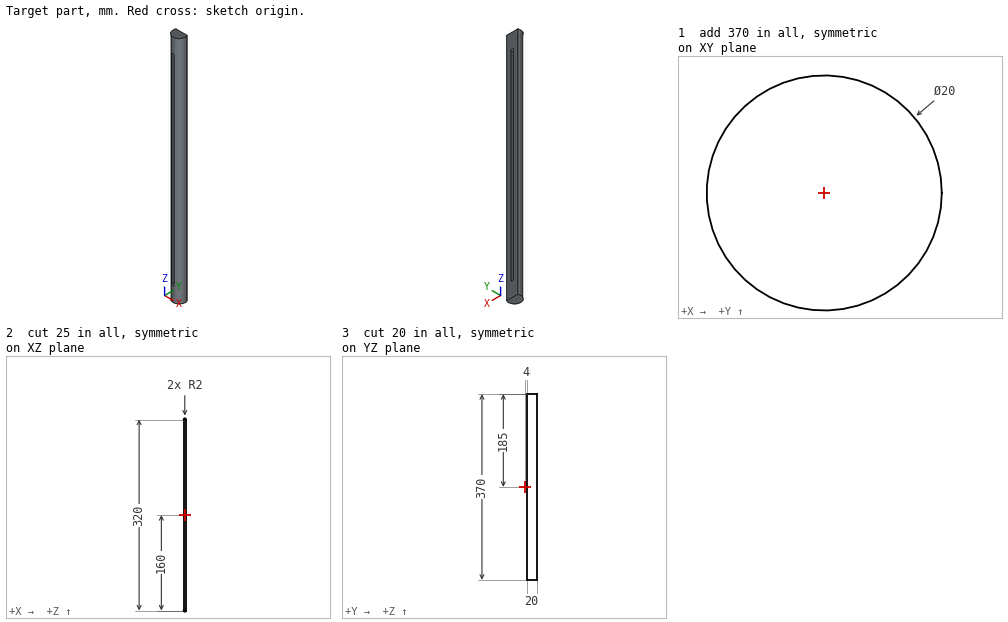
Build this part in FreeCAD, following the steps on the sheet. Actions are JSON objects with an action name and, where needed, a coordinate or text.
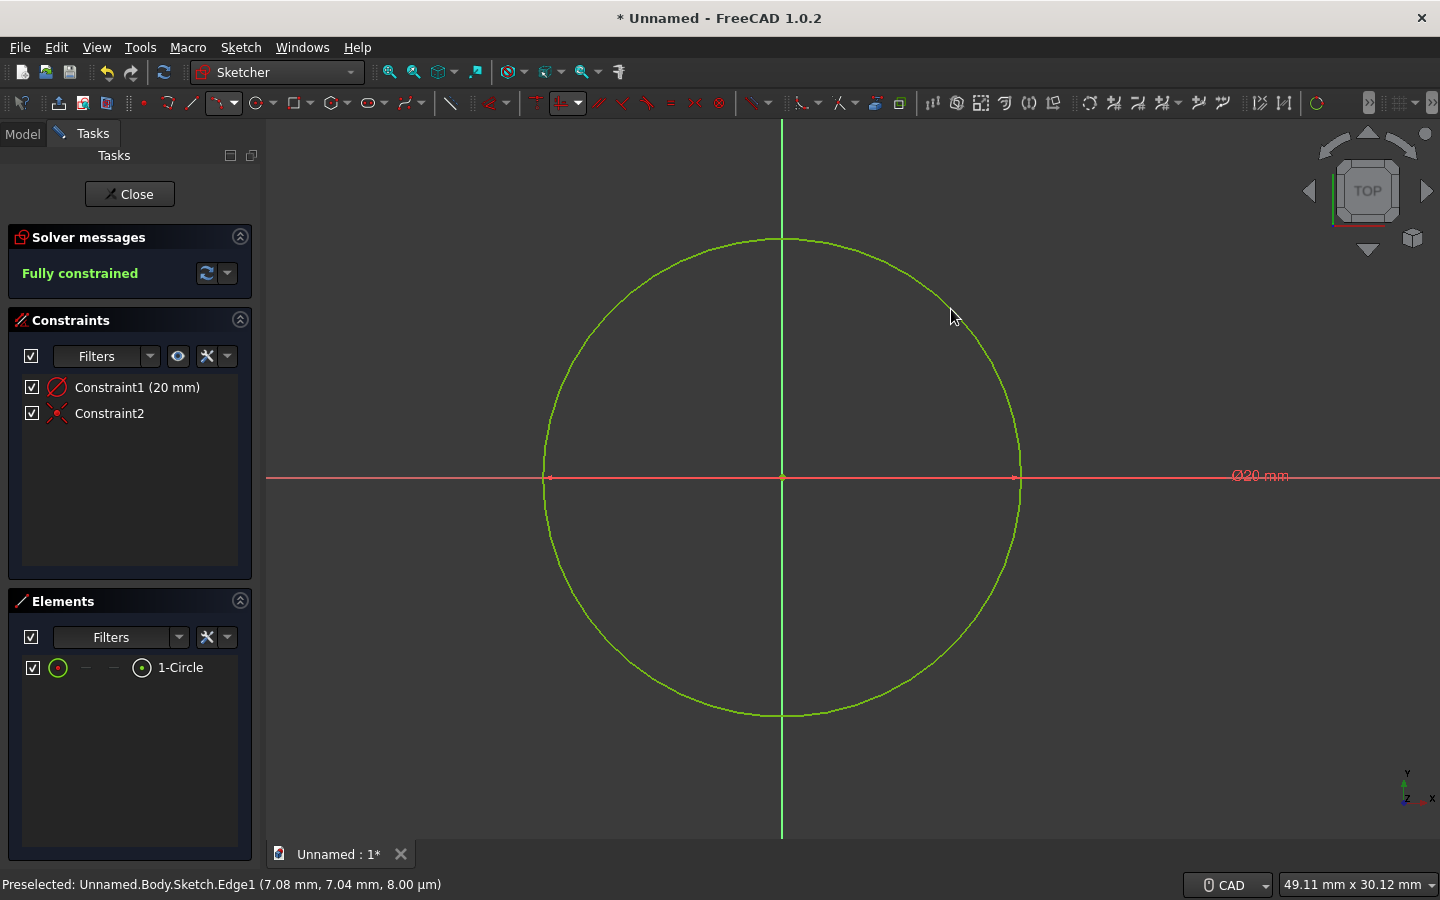
{"action": "left_click", "coordinate": [130, 194]}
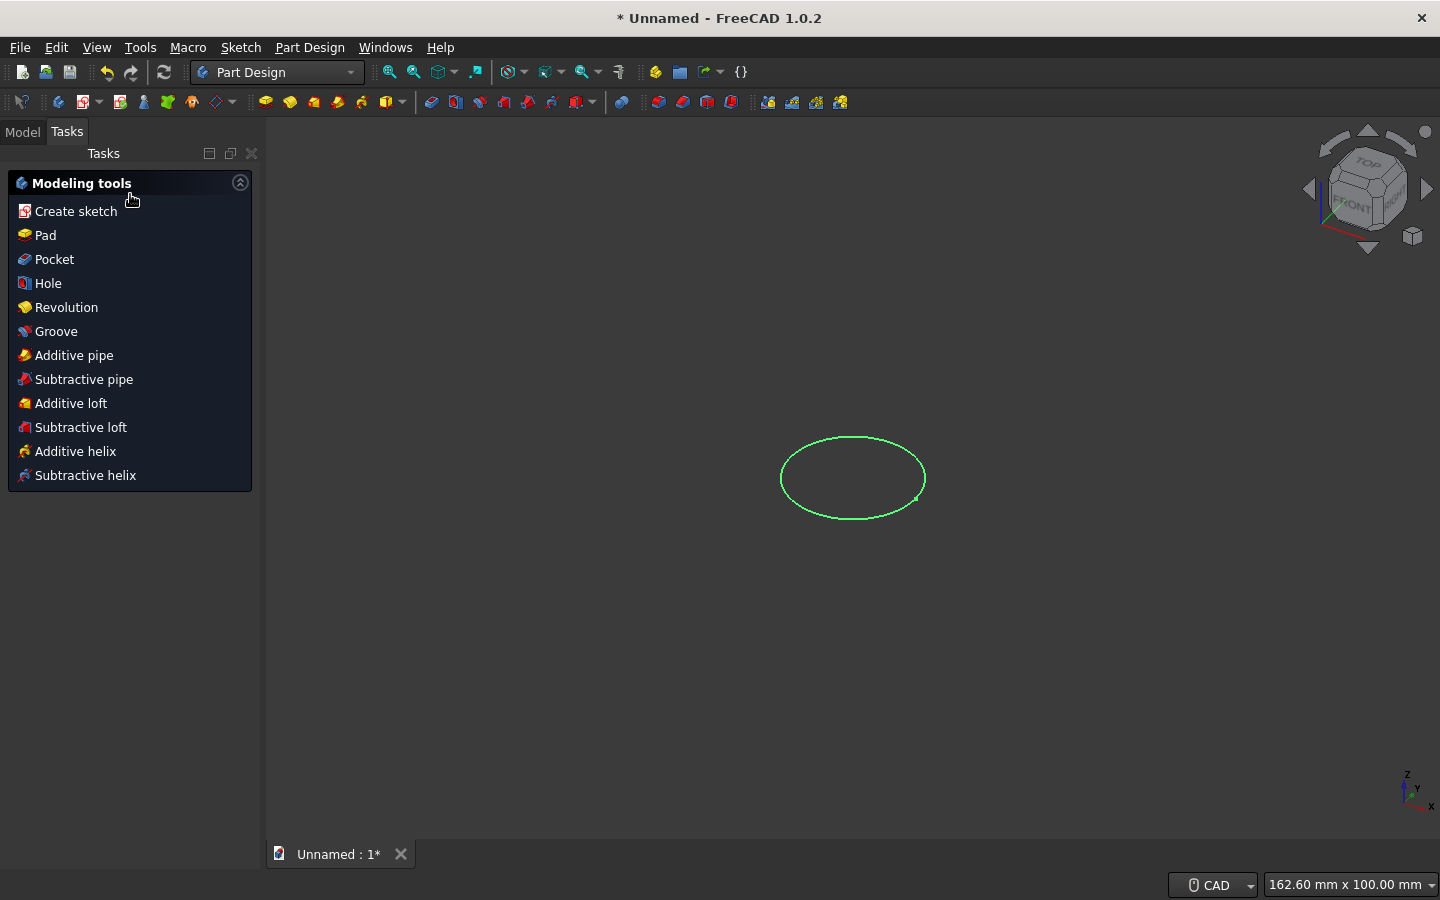
{"action": "left_click", "coordinate": [266, 102]}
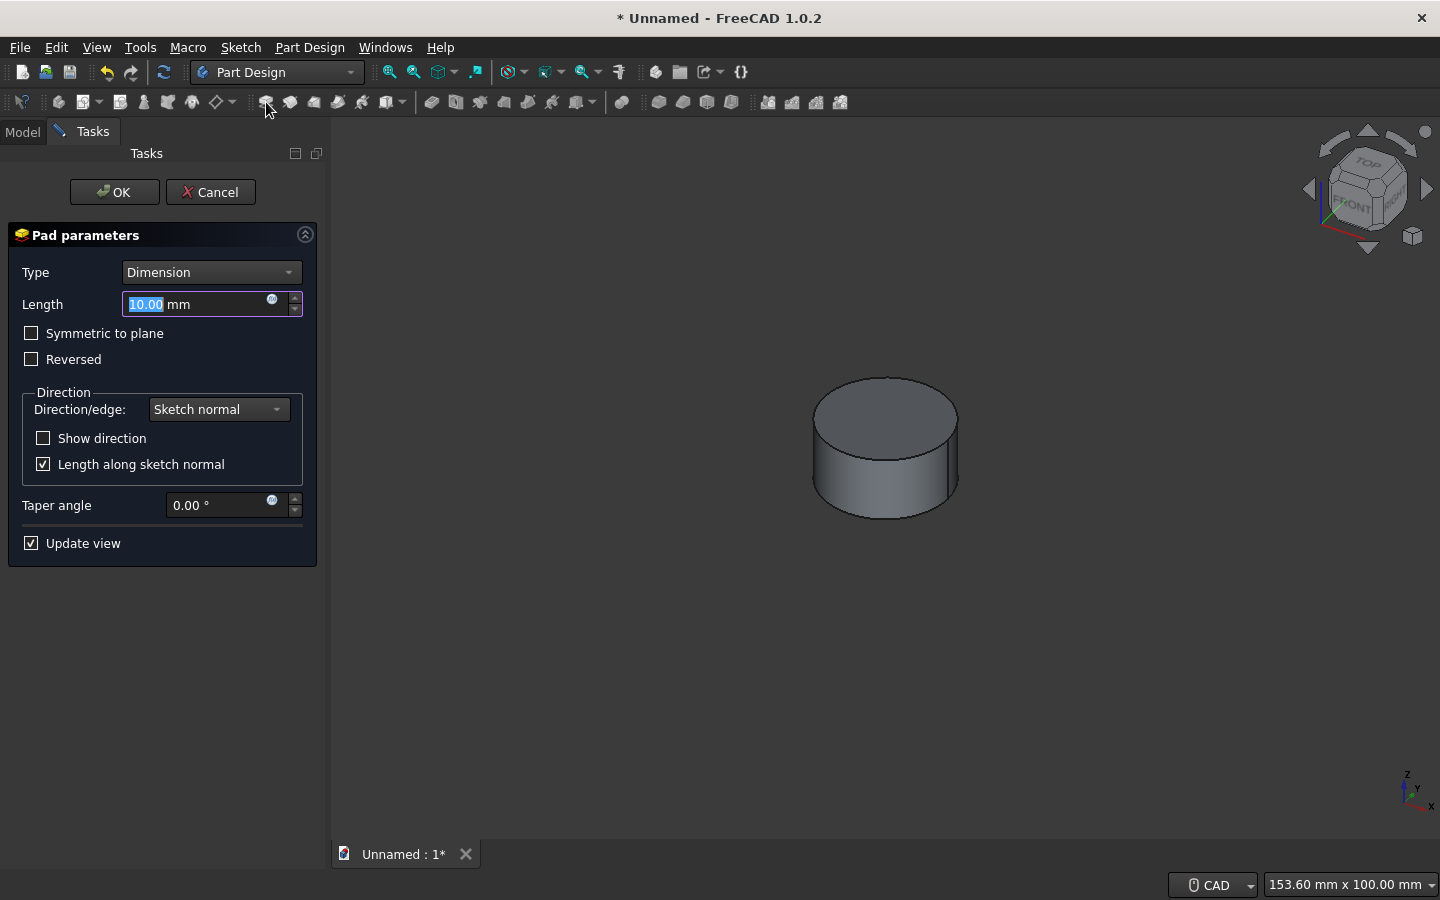
{"action": "type", "text": "370"}
{"action": "key", "text": "Tab"}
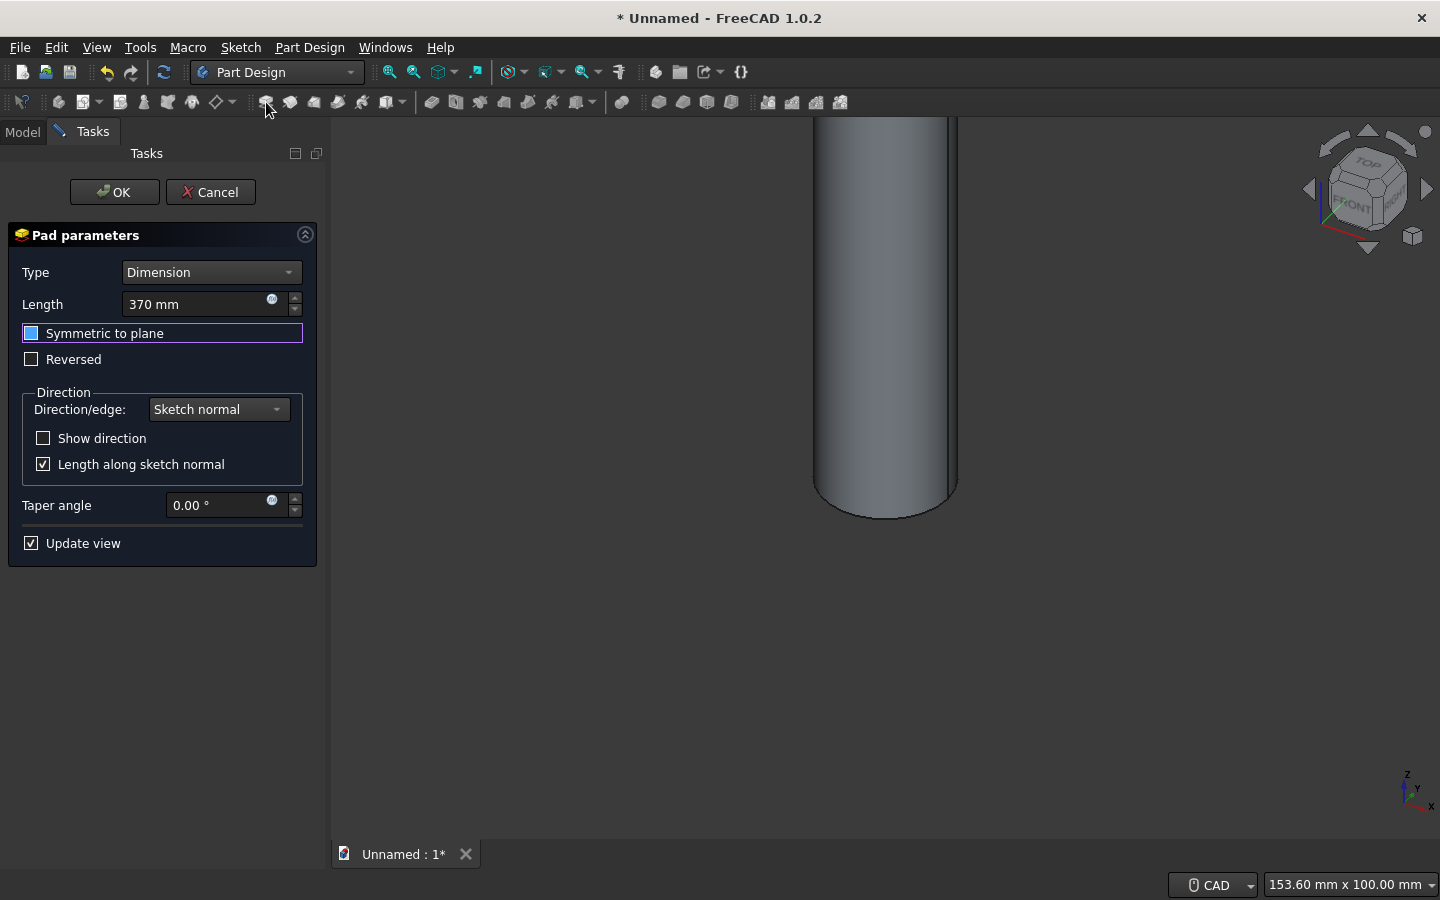
{"action": "left_click", "coordinate": [30, 333]}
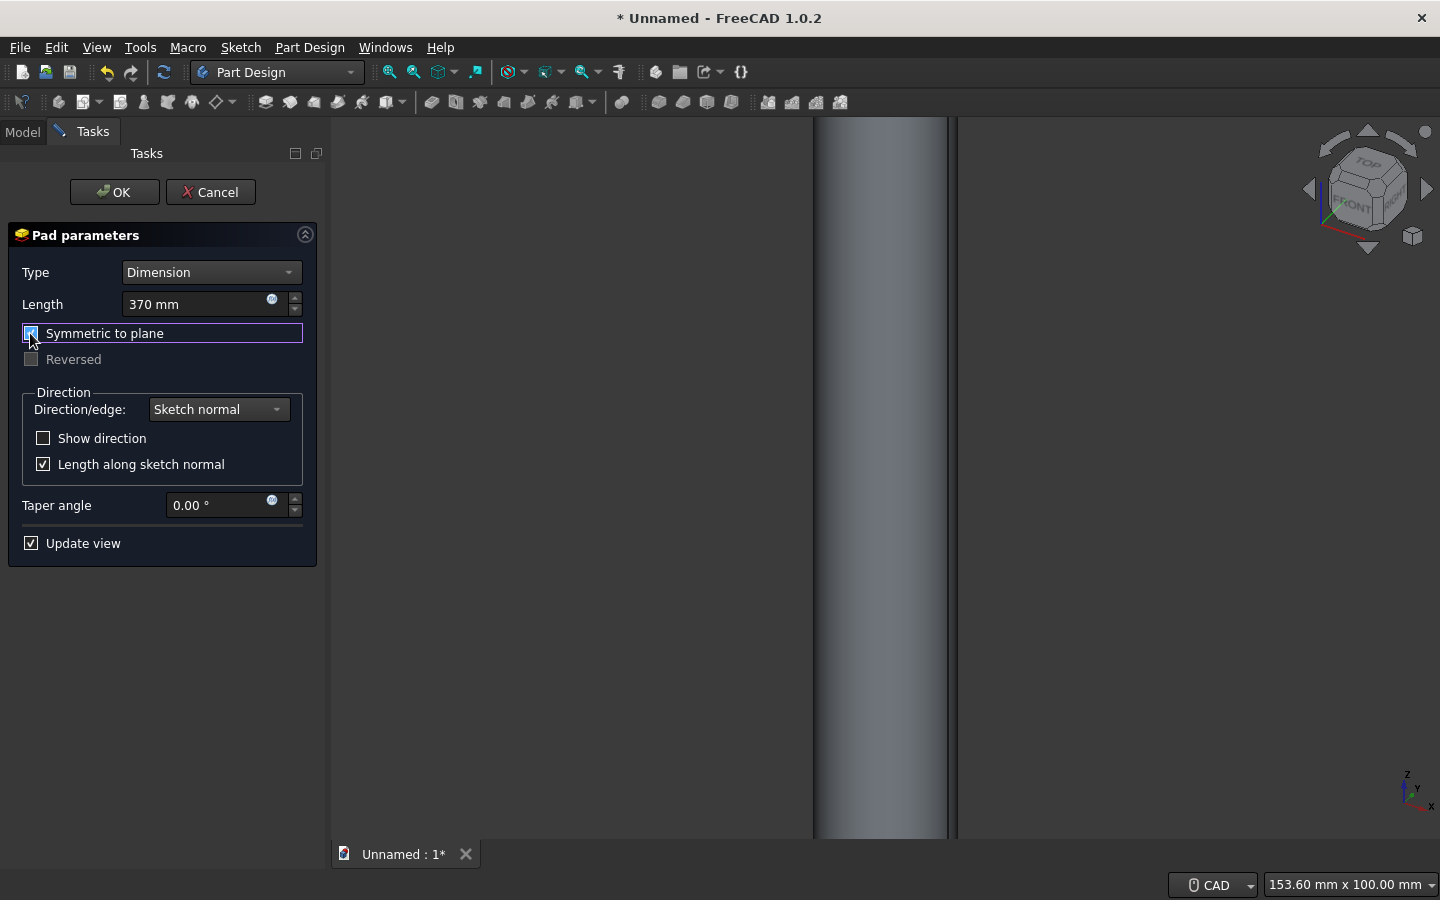
{"action": "left_click", "coordinate": [115, 192]}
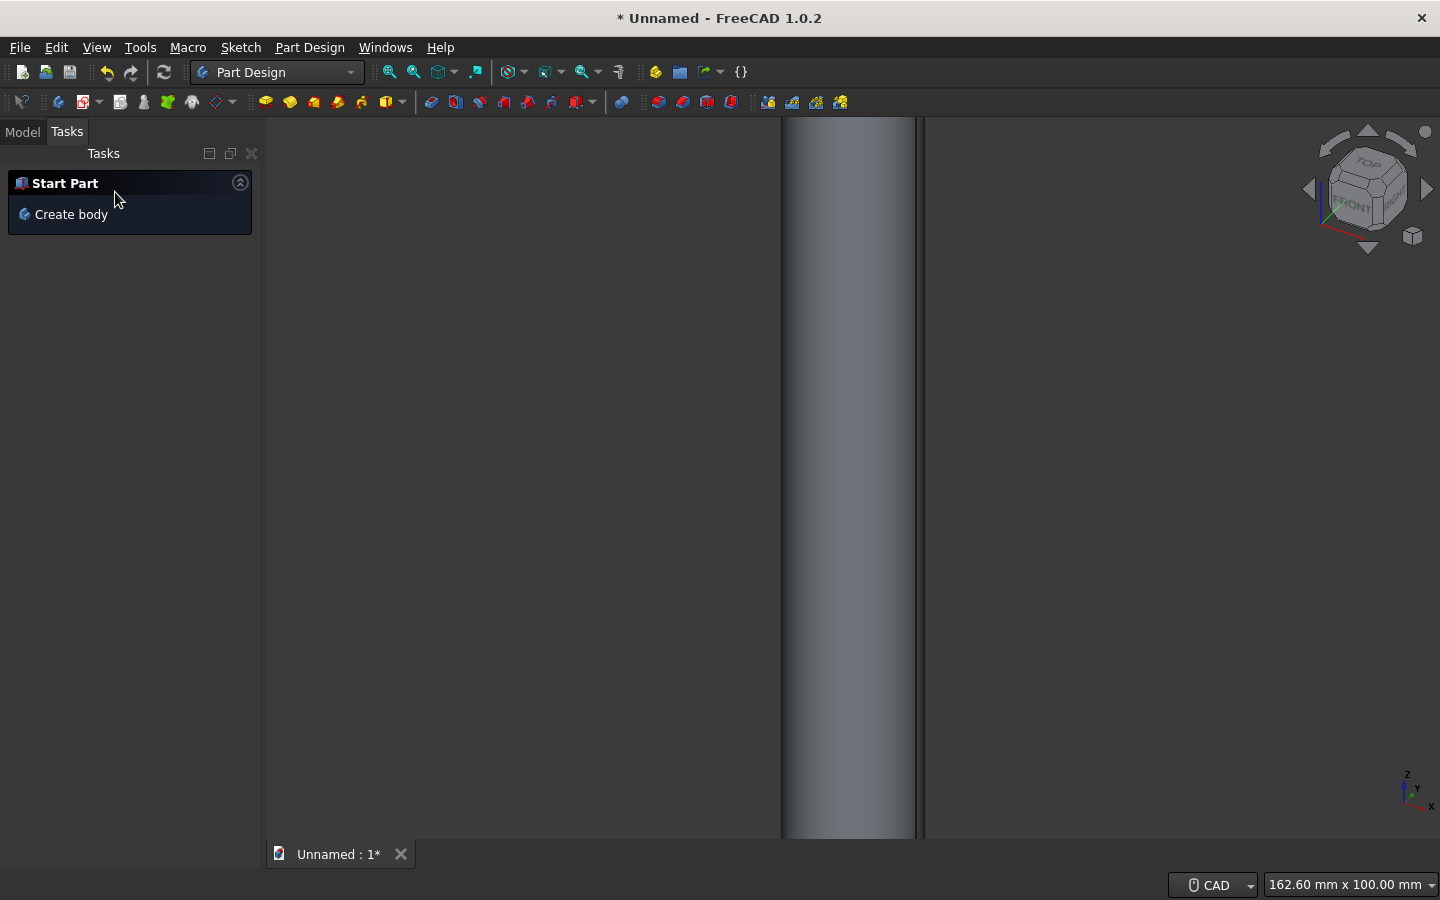
{"action": "left_click", "coordinate": [390, 72]}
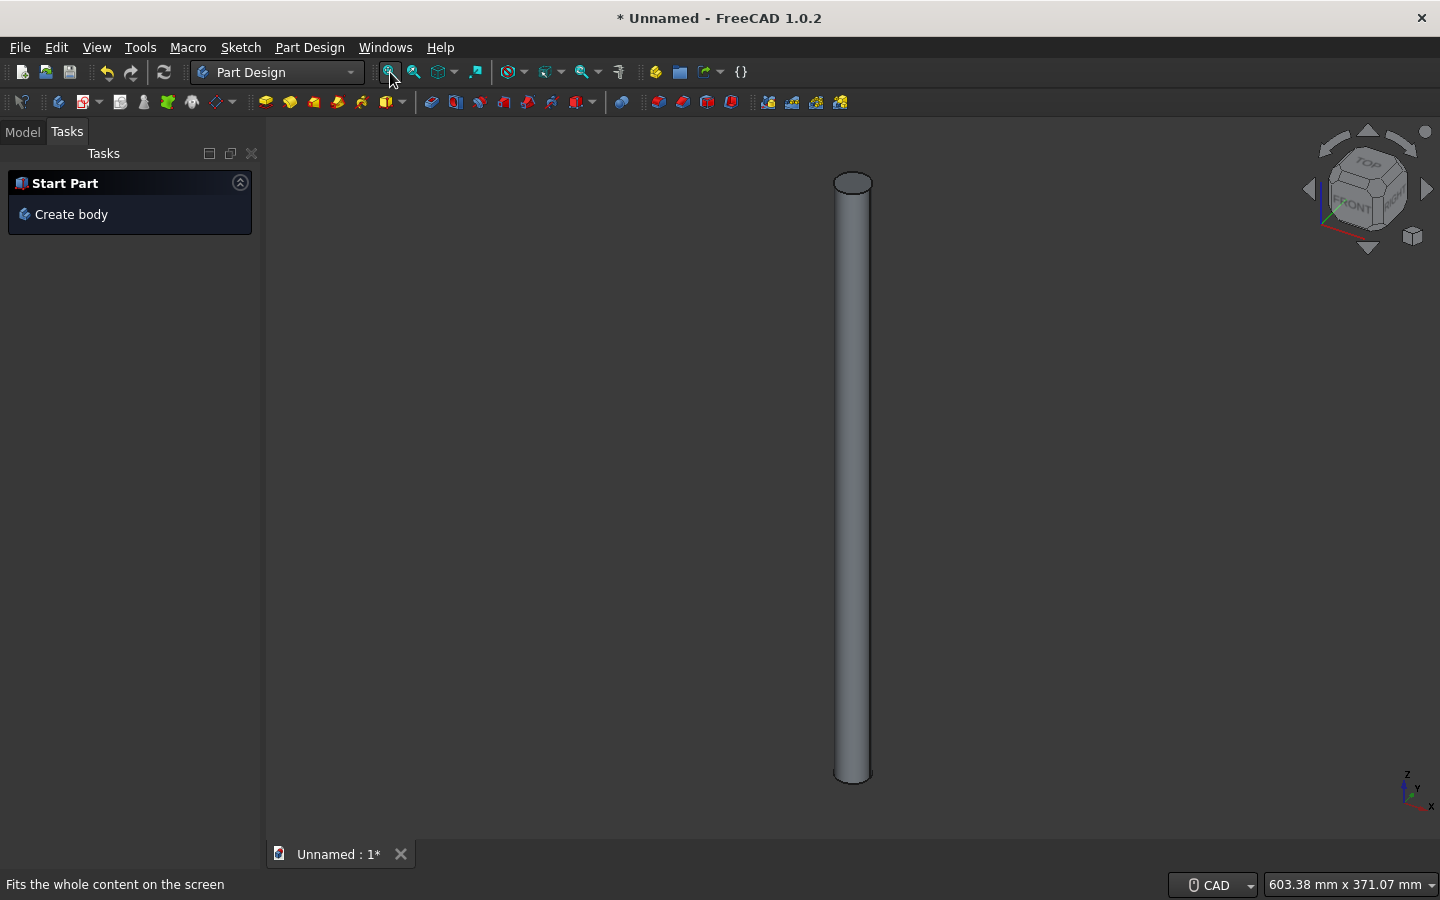
{"action": "left_click", "coordinate": [84, 102]}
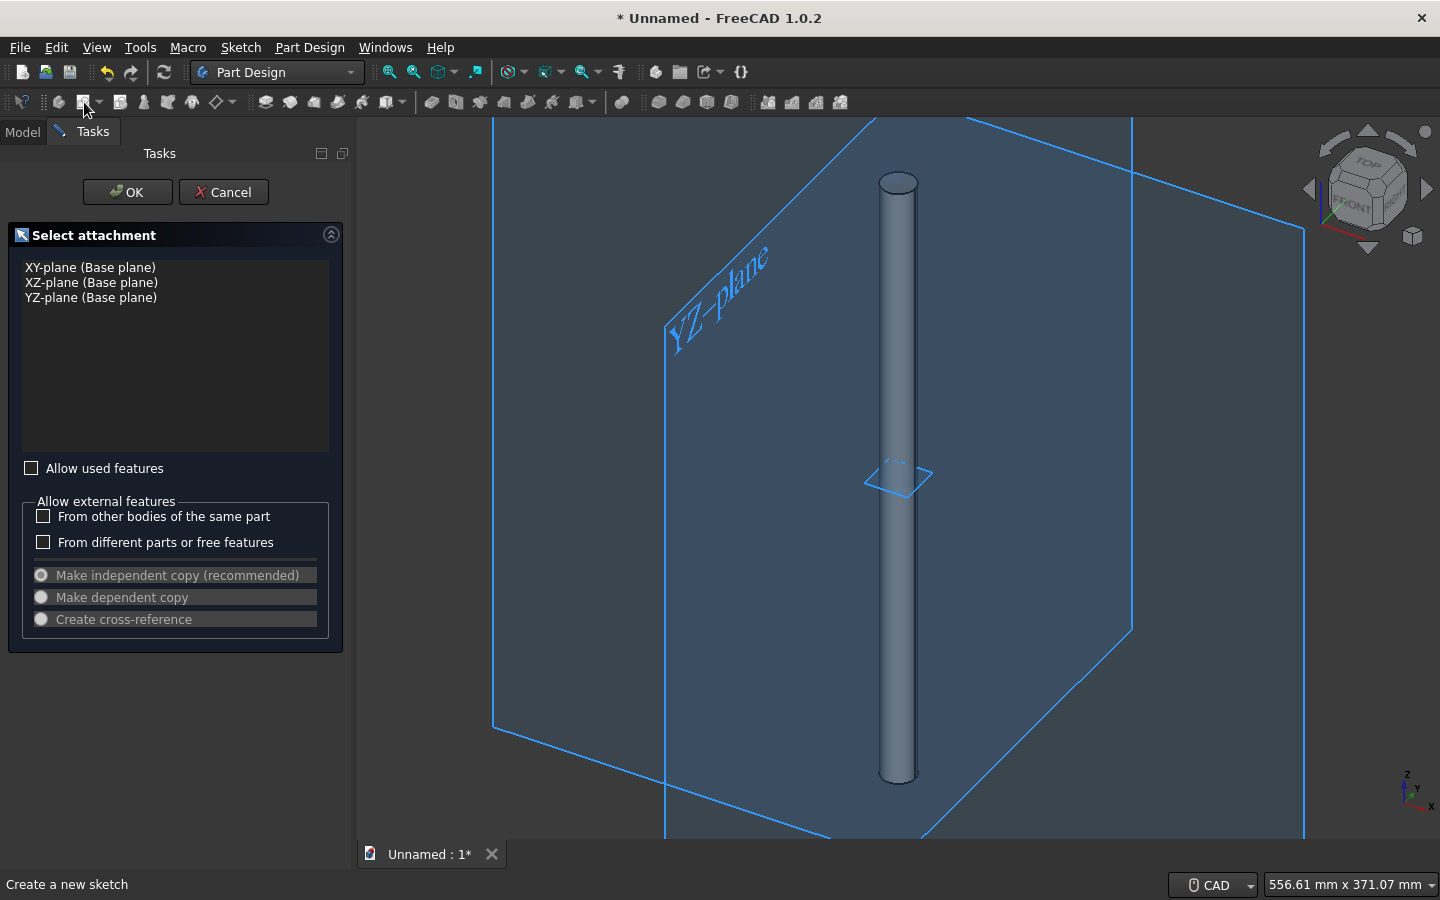
{"action": "left_click", "coordinate": [82, 282]}